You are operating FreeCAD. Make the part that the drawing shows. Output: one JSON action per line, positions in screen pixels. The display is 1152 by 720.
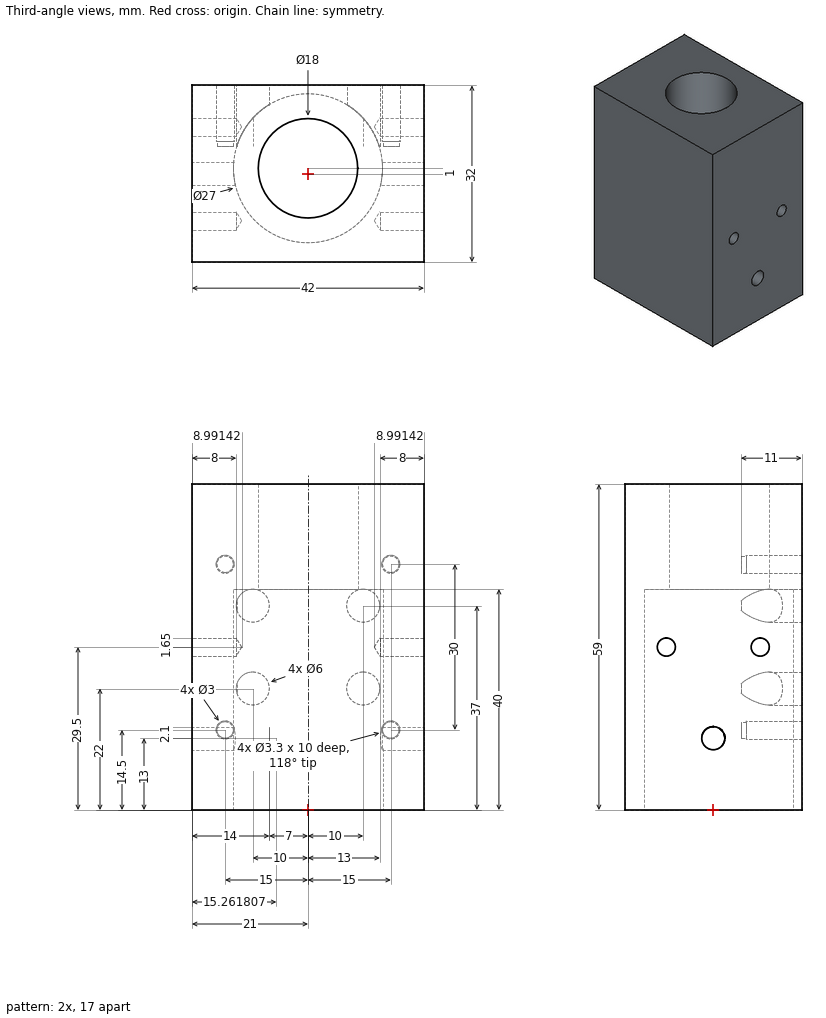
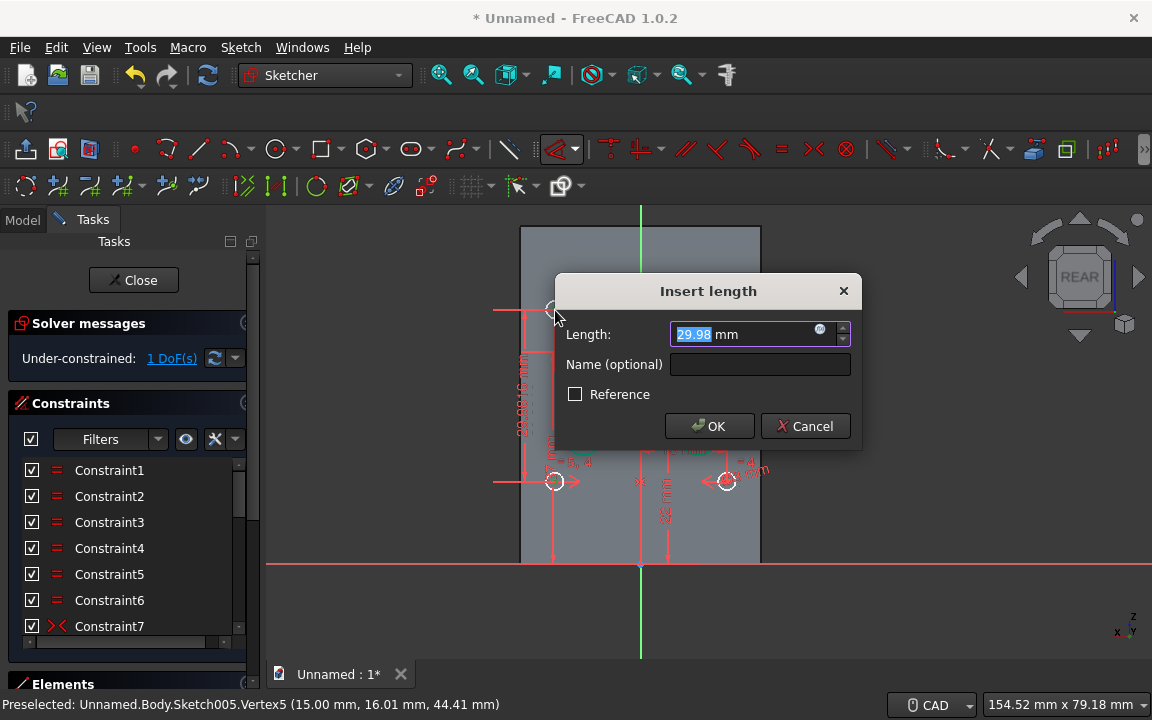
{"action": "type", "text": "30"}
{"action": "key", "text": "Return"}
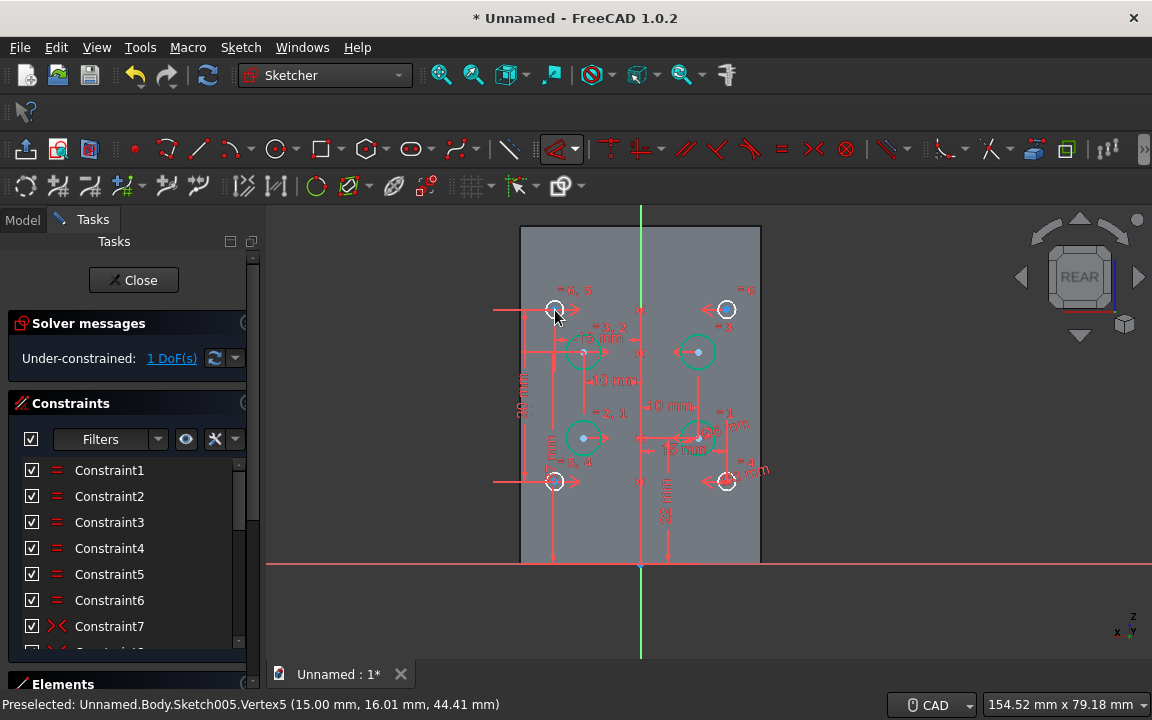
{"action": "left_click", "coordinate": [727, 482]}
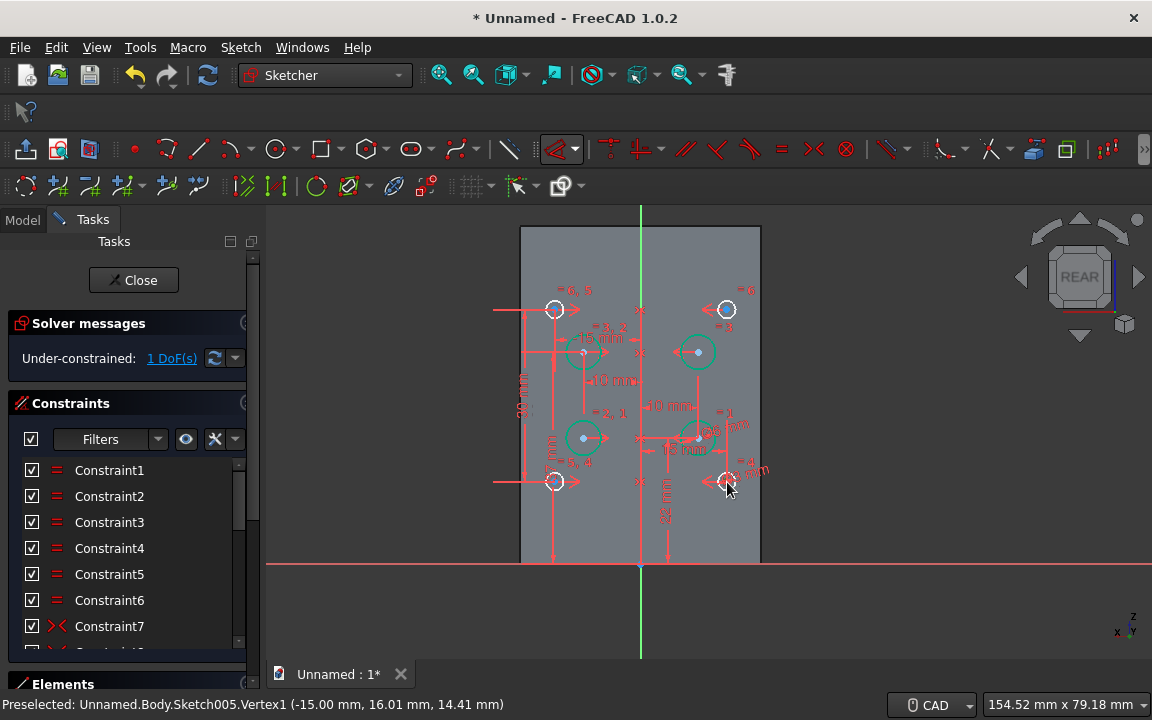
{"action": "left_click", "coordinate": [578, 150]}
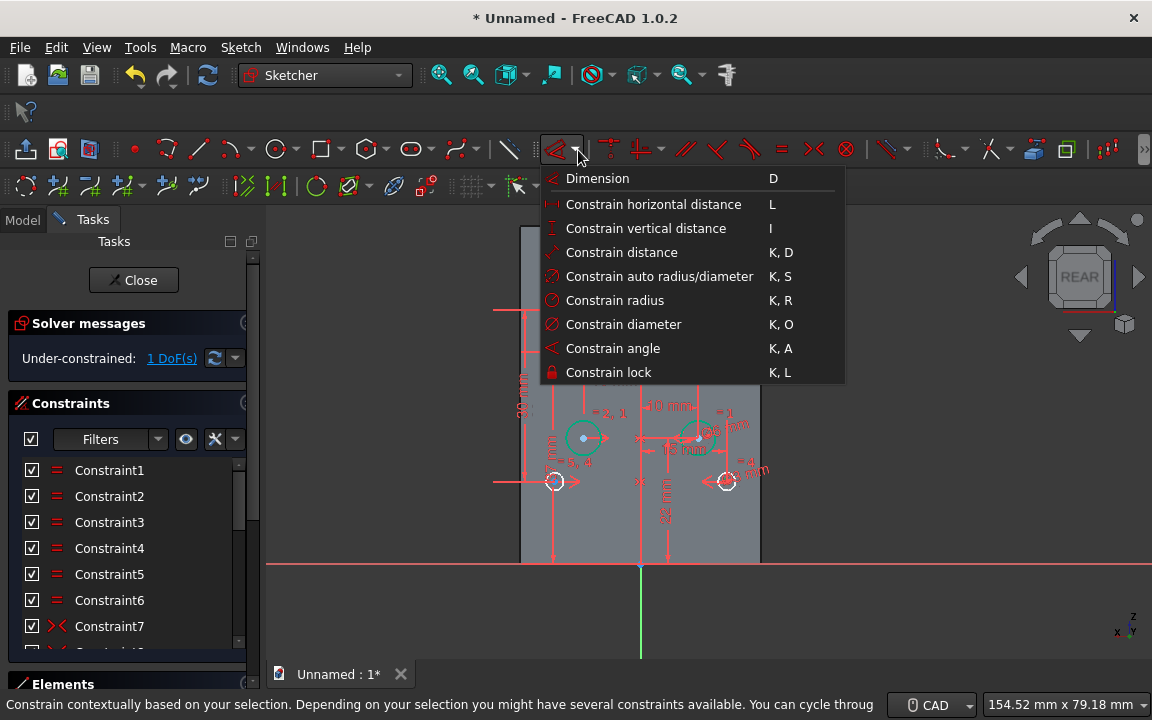
{"action": "left_click", "coordinate": [693, 228]}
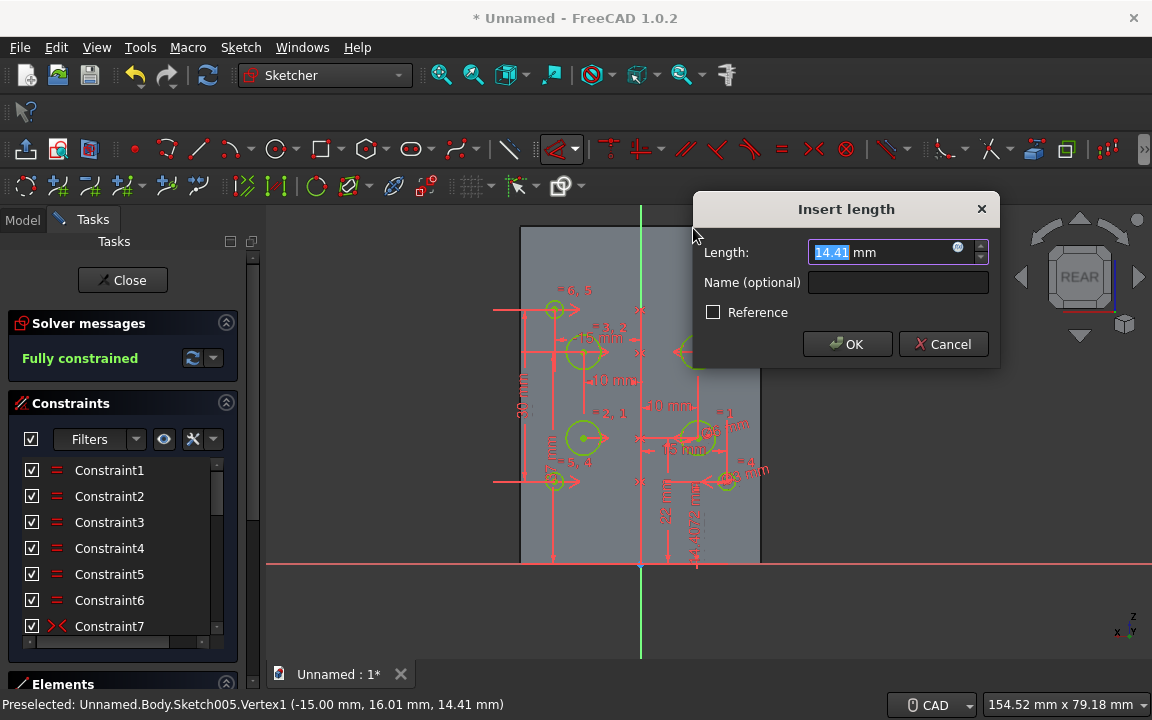
{"action": "type", "text": "14.5"}
{"action": "key", "text": "Return"}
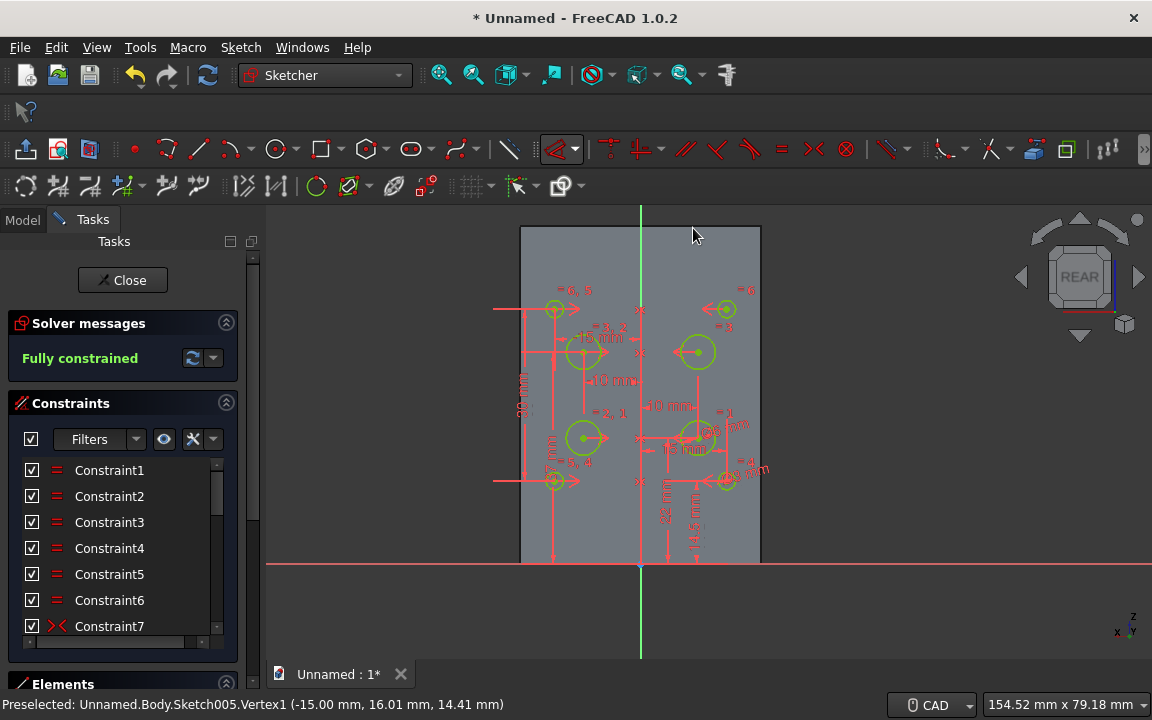
{"action": "left_click", "coordinate": [123, 280]}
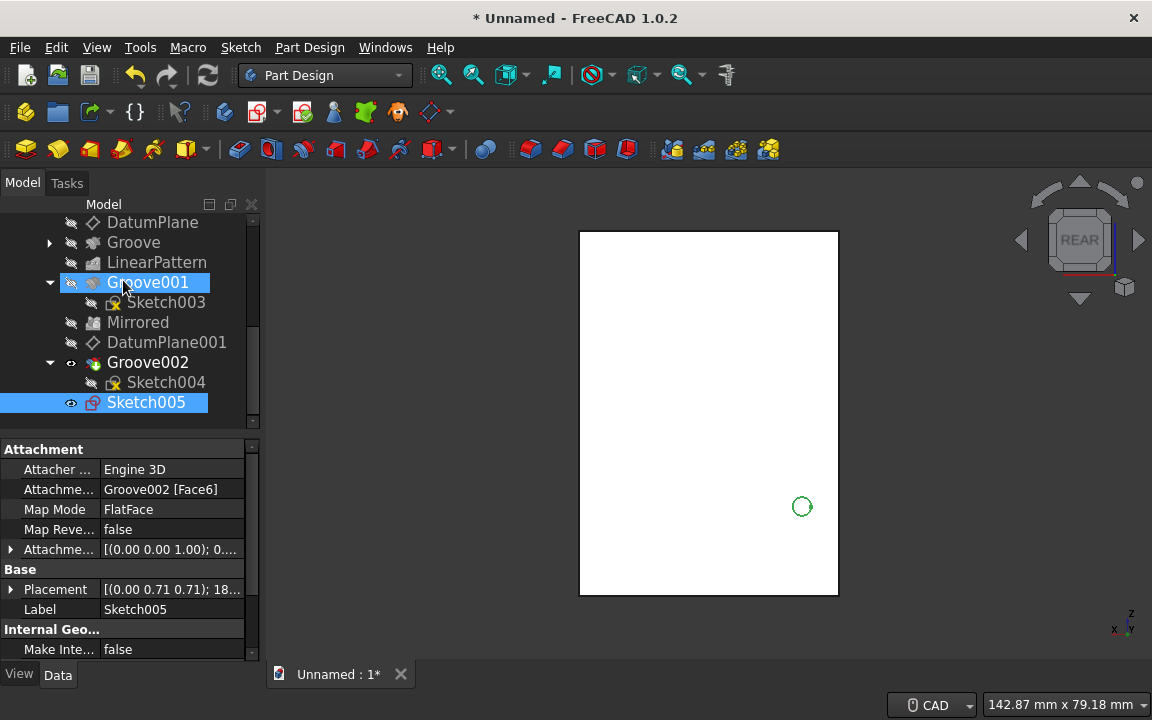
{"action": "left_click", "coordinate": [240, 150]}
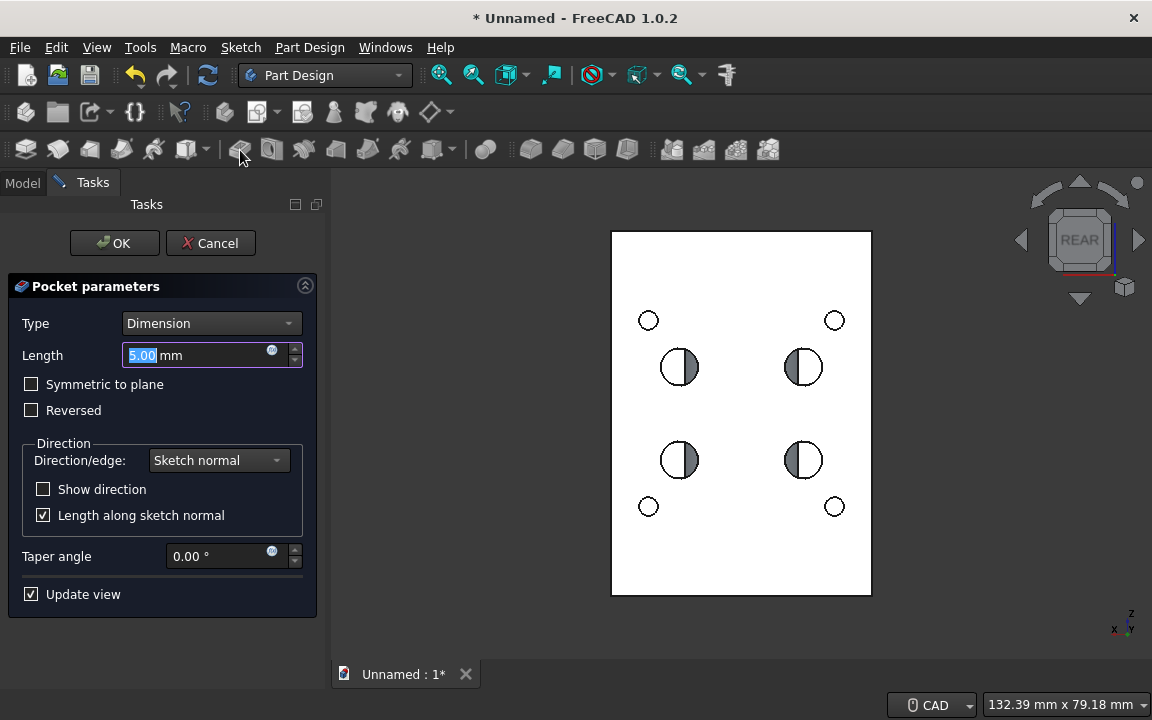
{"action": "type", "text": "11"}
{"action": "key", "text": "Tab"}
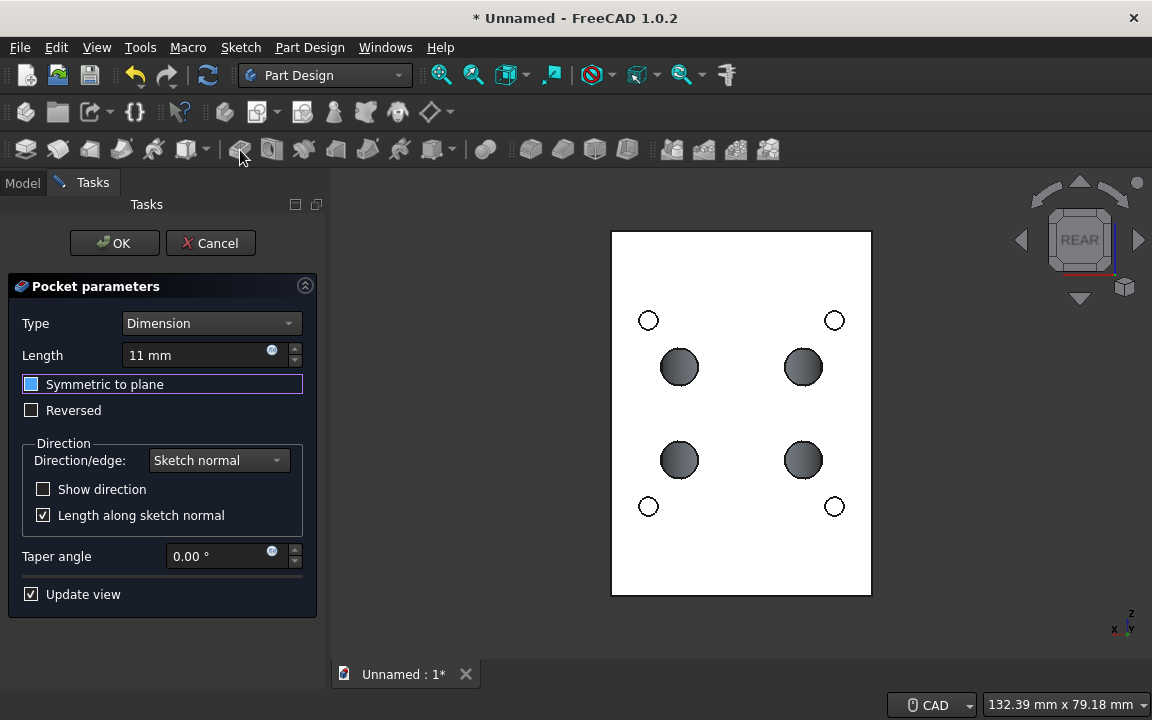
{"action": "left_click", "coordinate": [115, 243]}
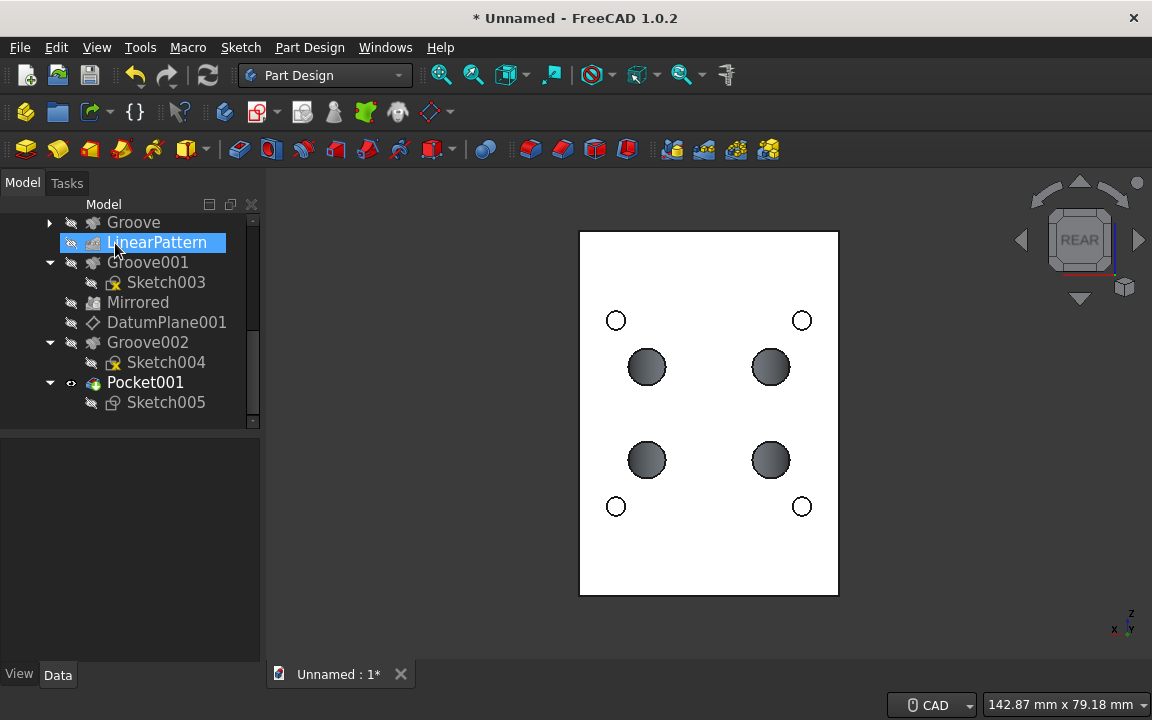
{"action": "left_click", "coordinate": [709, 308]}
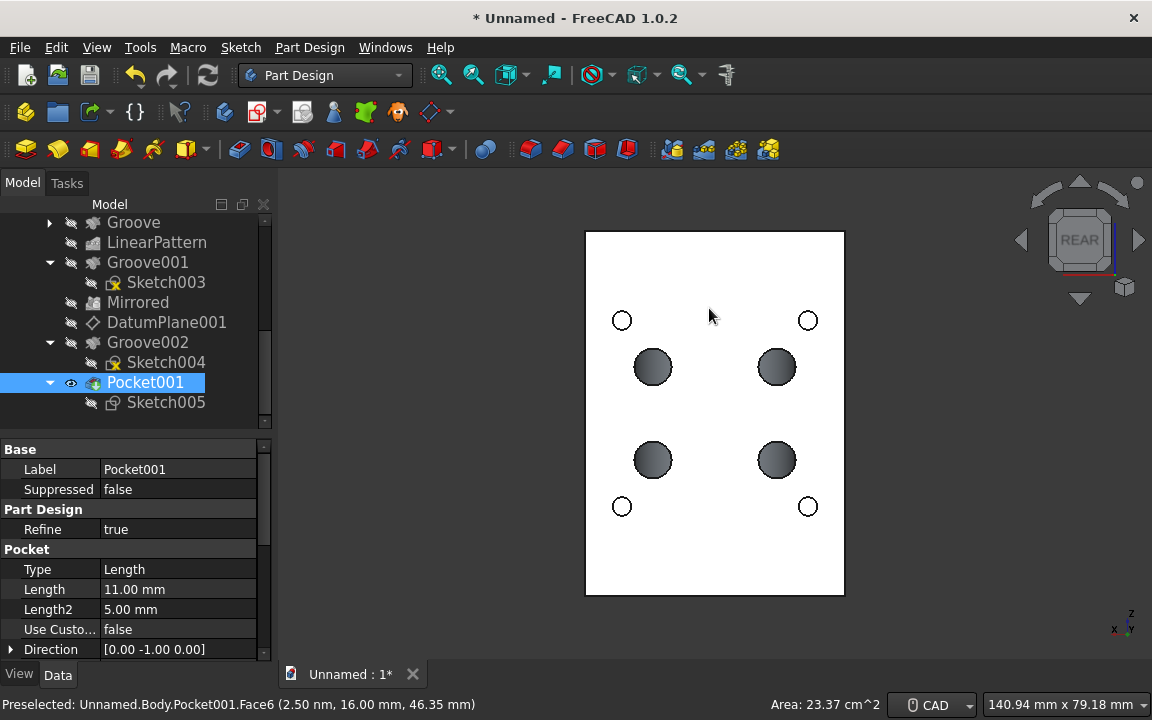
{"action": "left_click", "coordinate": [258, 112]}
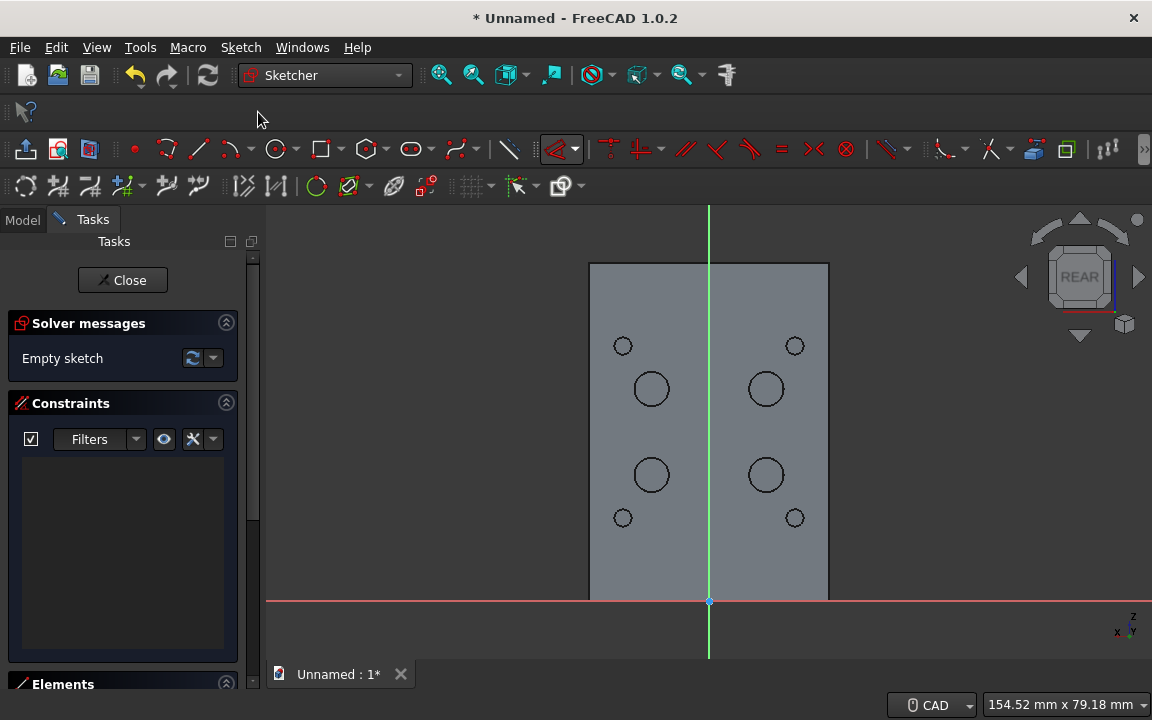
{"action": "left_click", "coordinate": [276, 150]}